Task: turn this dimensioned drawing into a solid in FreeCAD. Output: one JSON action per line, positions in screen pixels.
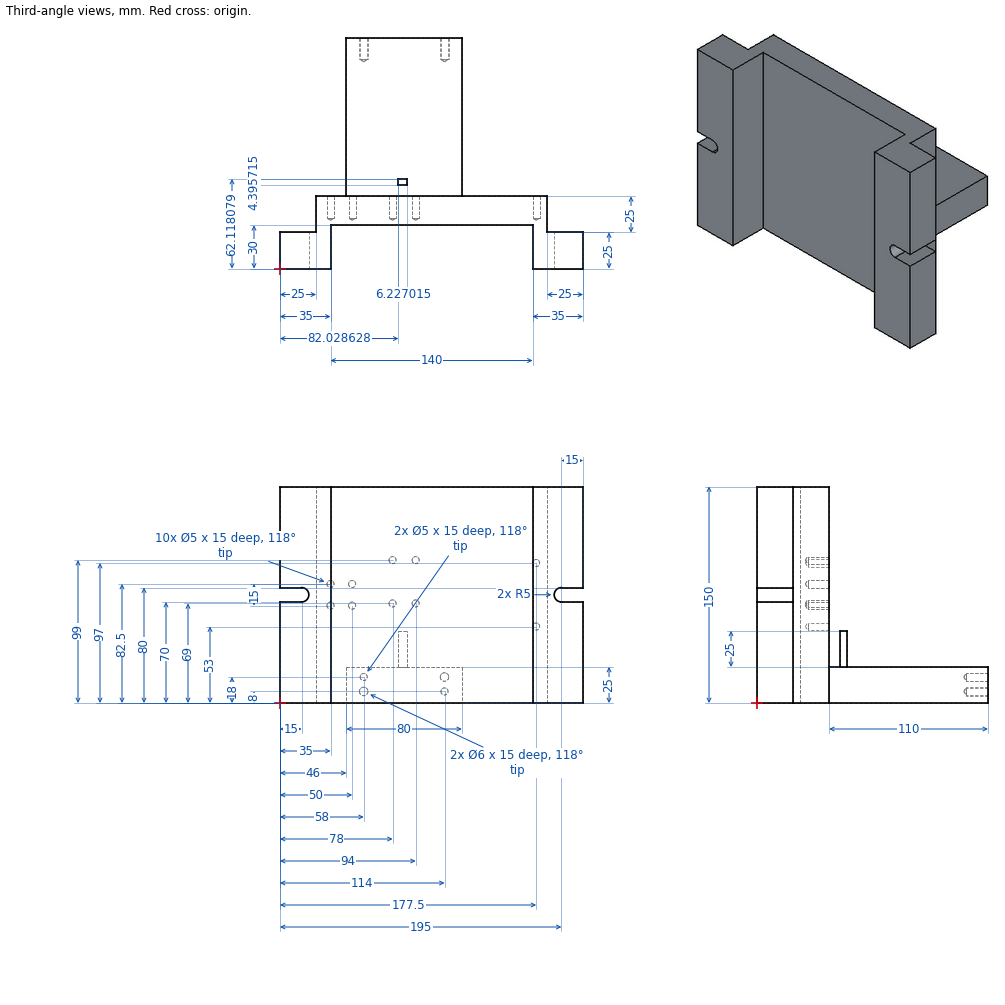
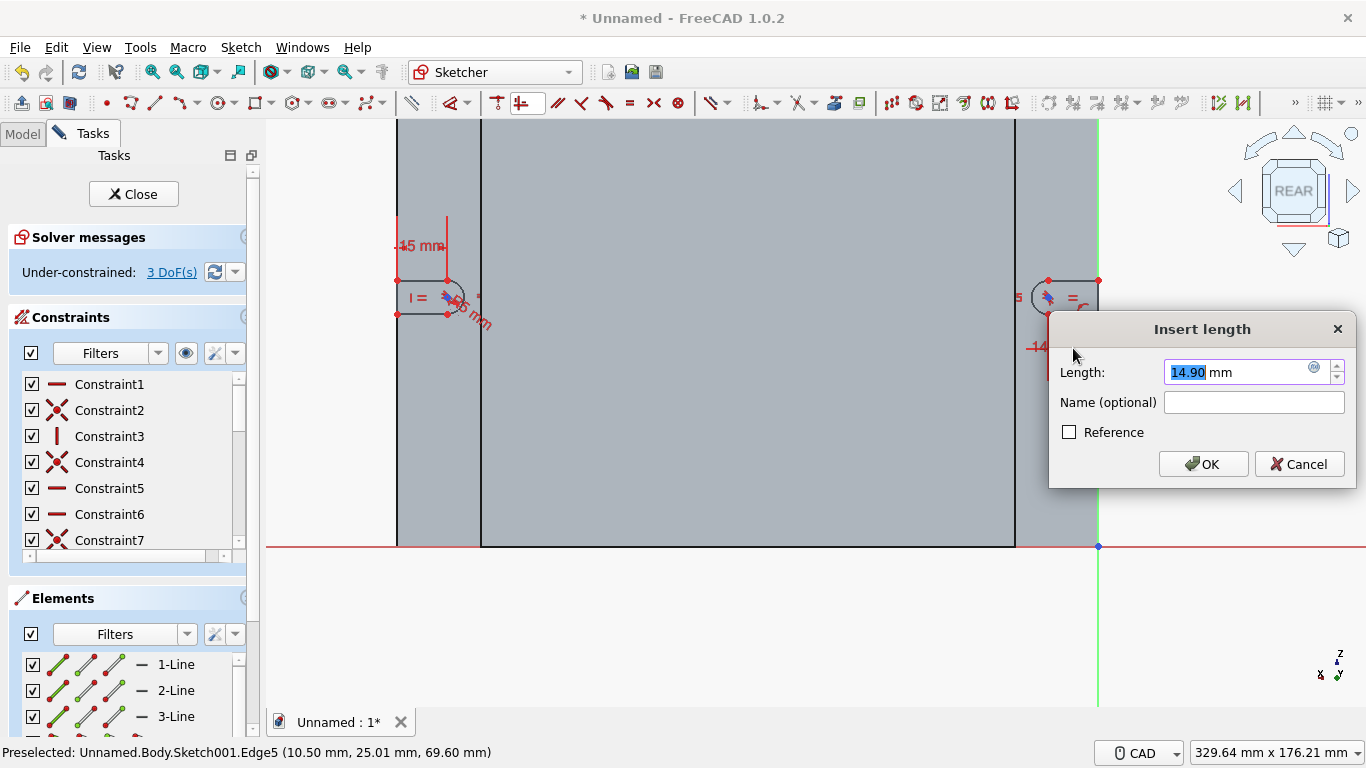
{"action": "type", "text": "15"}
{"action": "key", "text": "Return"}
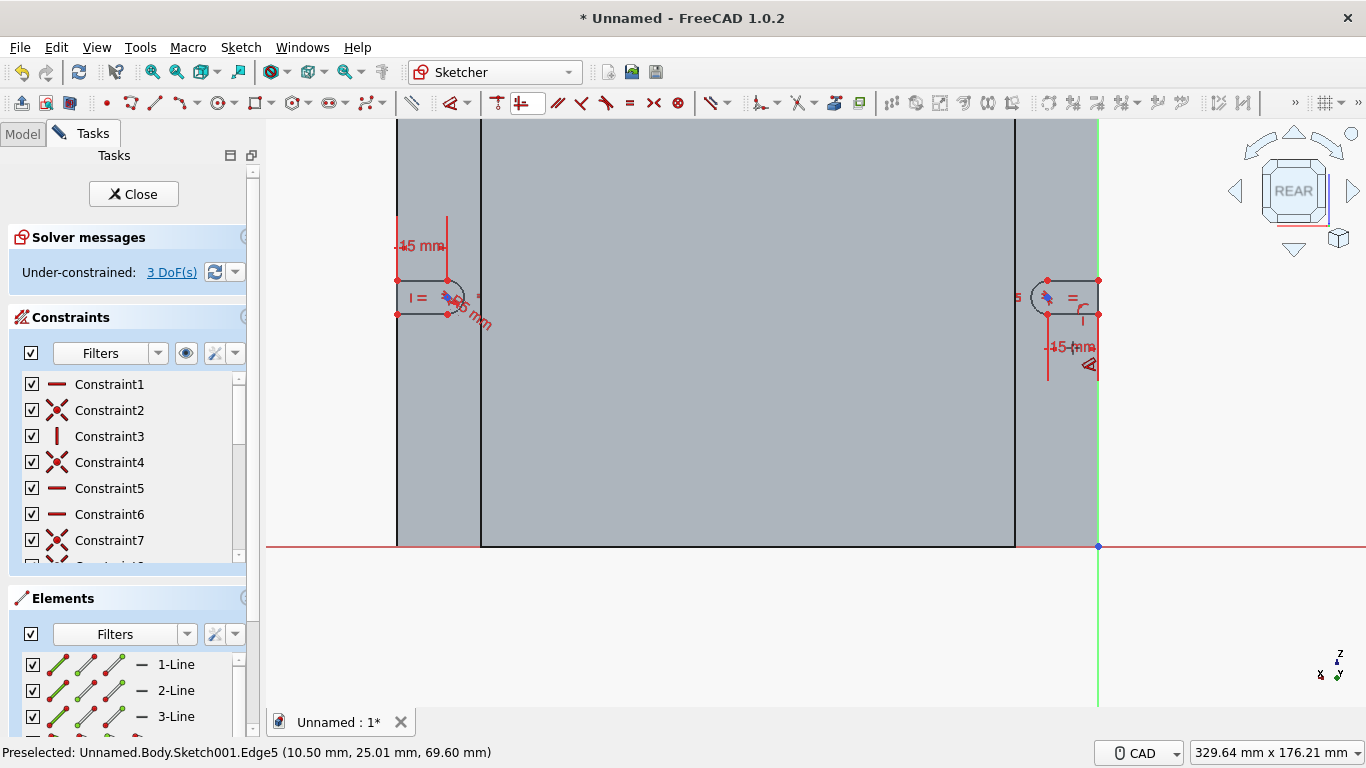
{"action": "left_click", "coordinate": [447, 281]}
{"action": "left_click", "coordinate": [1132, 414]}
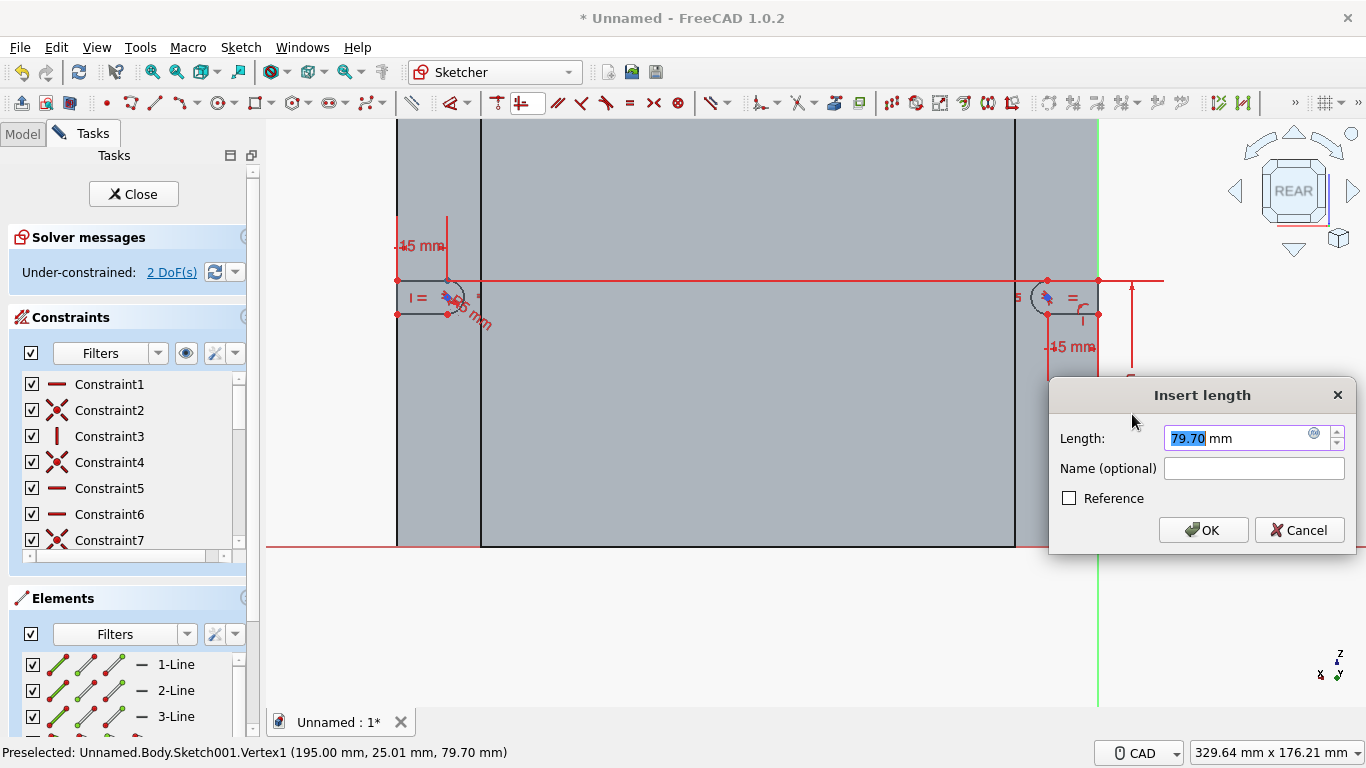
{"action": "type", "text": "80"}
{"action": "key", "text": "Return"}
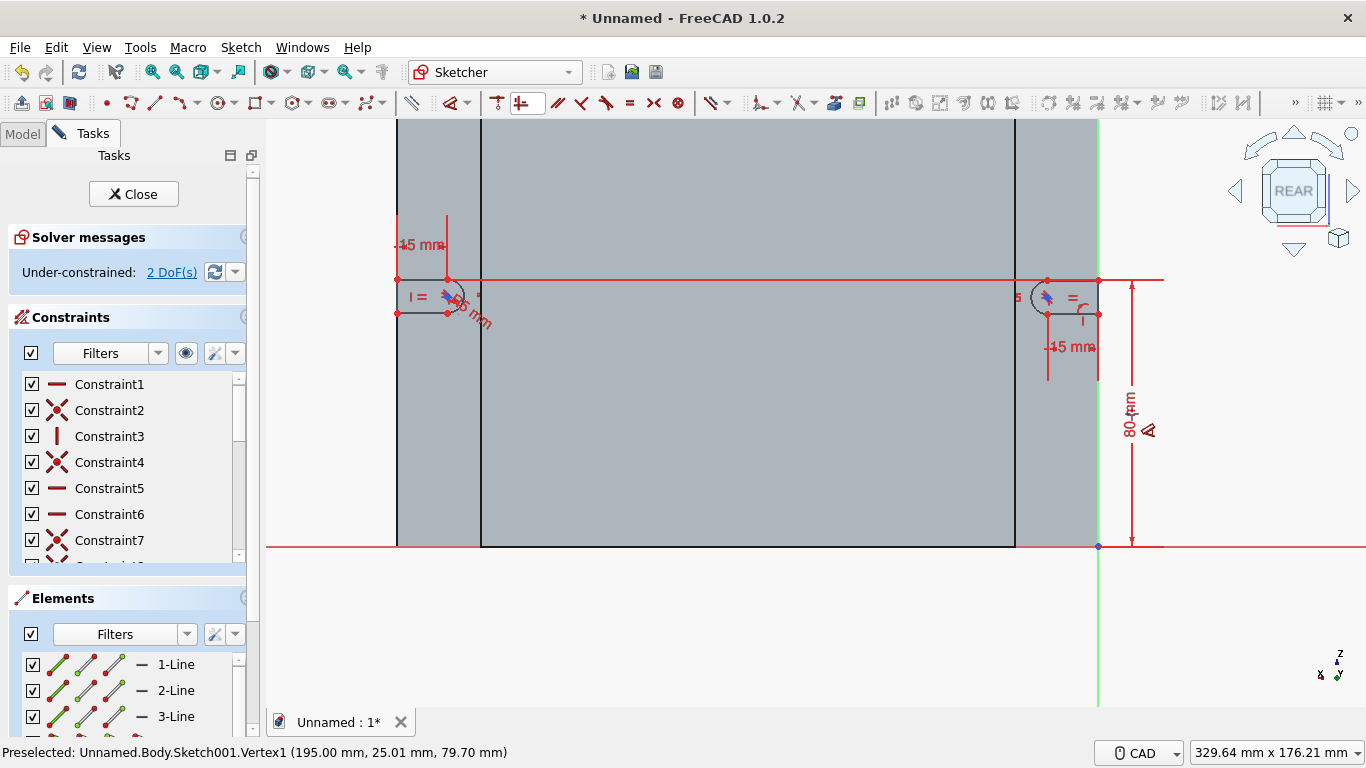
{"action": "left_click", "coordinate": [1048, 314]}
{"action": "left_click", "coordinate": [1132, 377]}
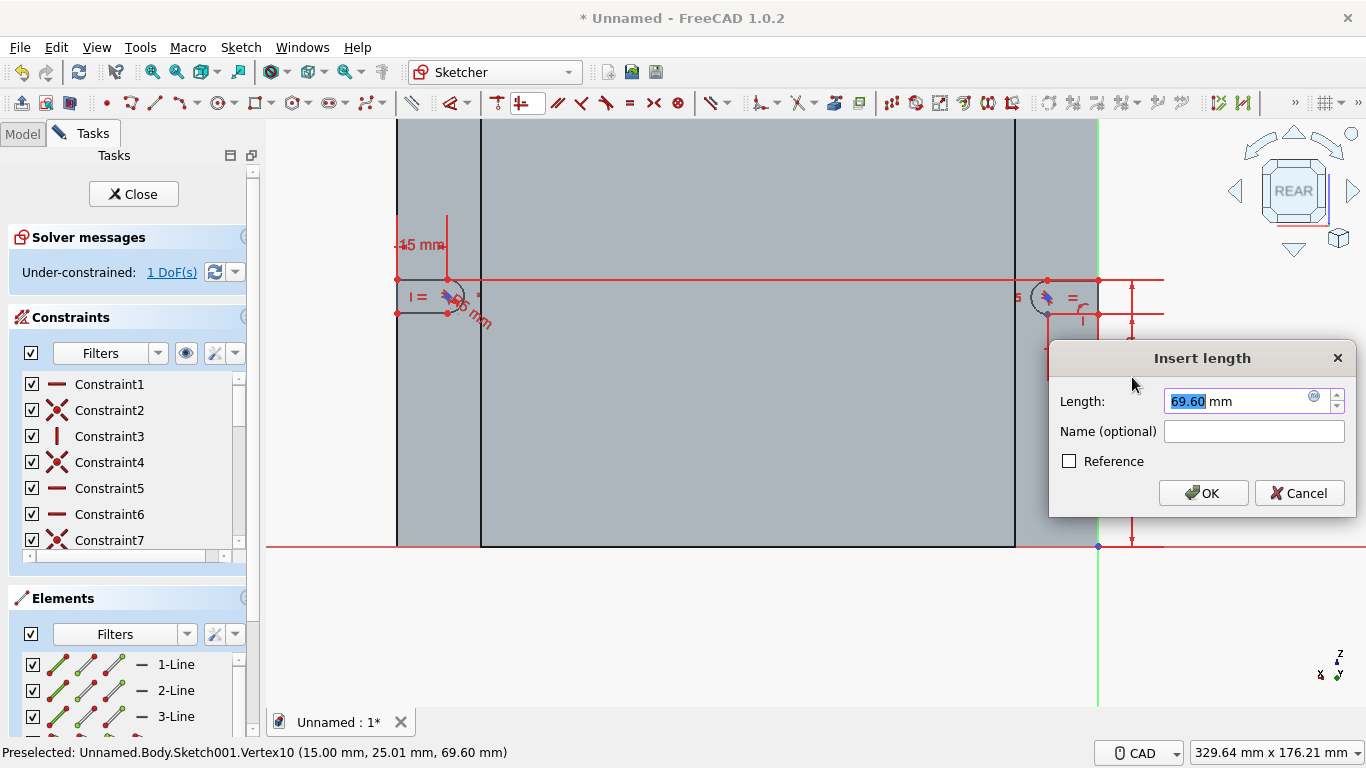
{"action": "type", "text": "70"}
{"action": "key", "text": "Return"}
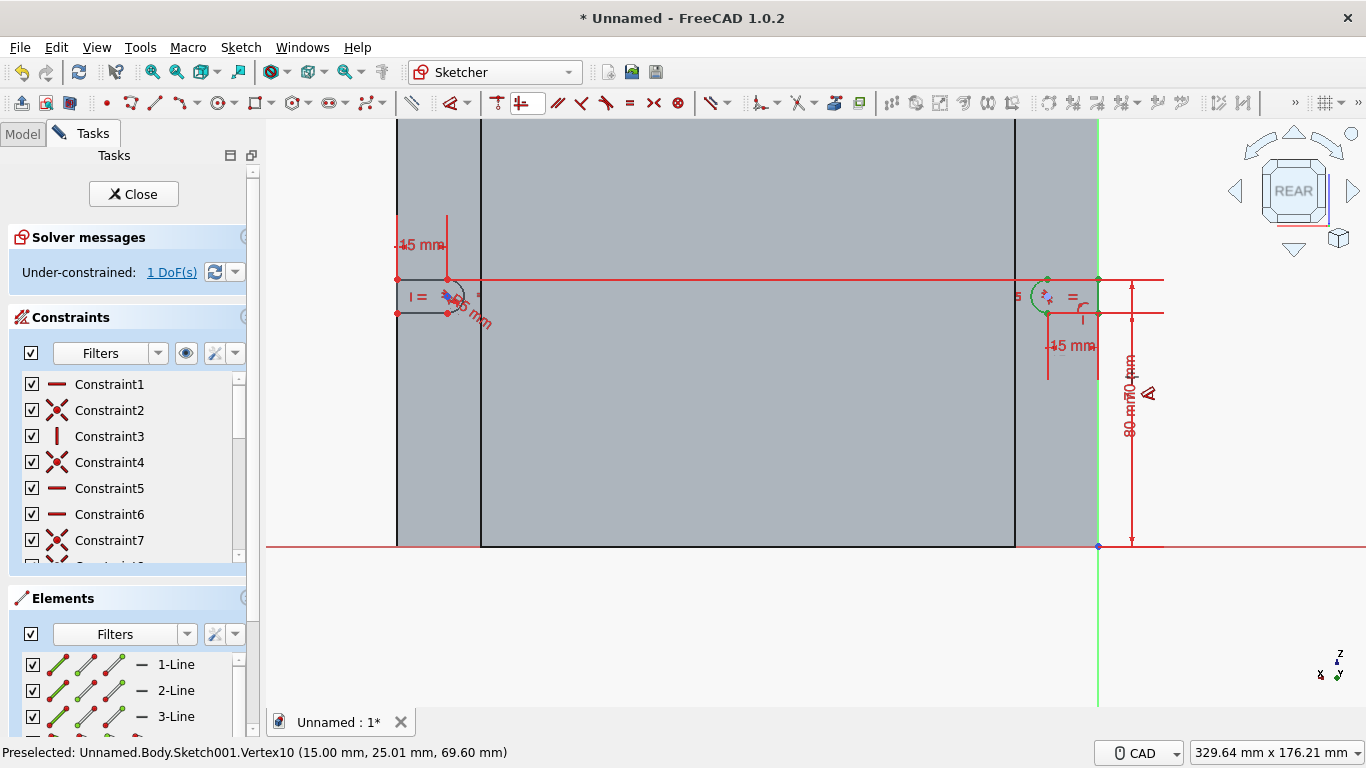
{"action": "left_click", "coordinate": [447, 280]}
{"action": "left_click", "coordinate": [773, 581]}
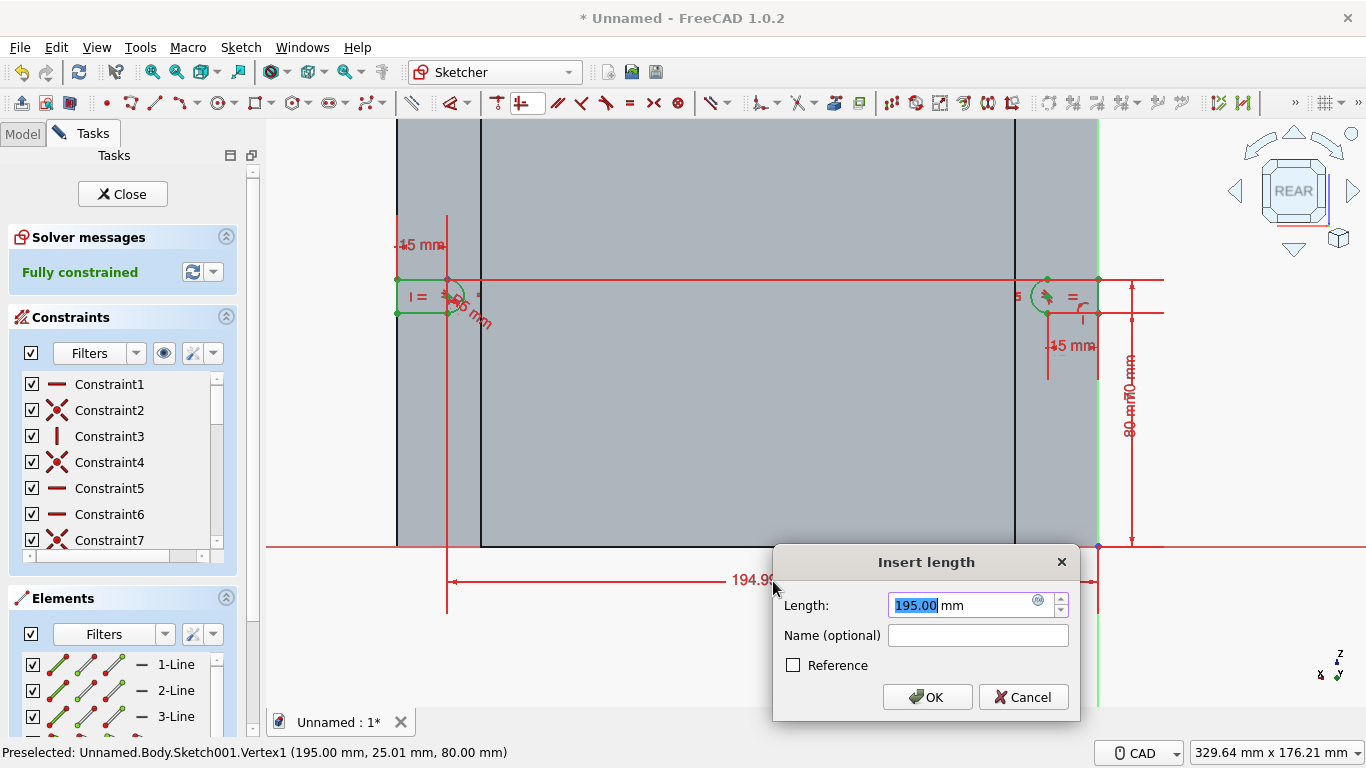
{"action": "type", "text": "195"}
{"action": "key", "text": "Return"}
{"action": "key", "text": "Escape"}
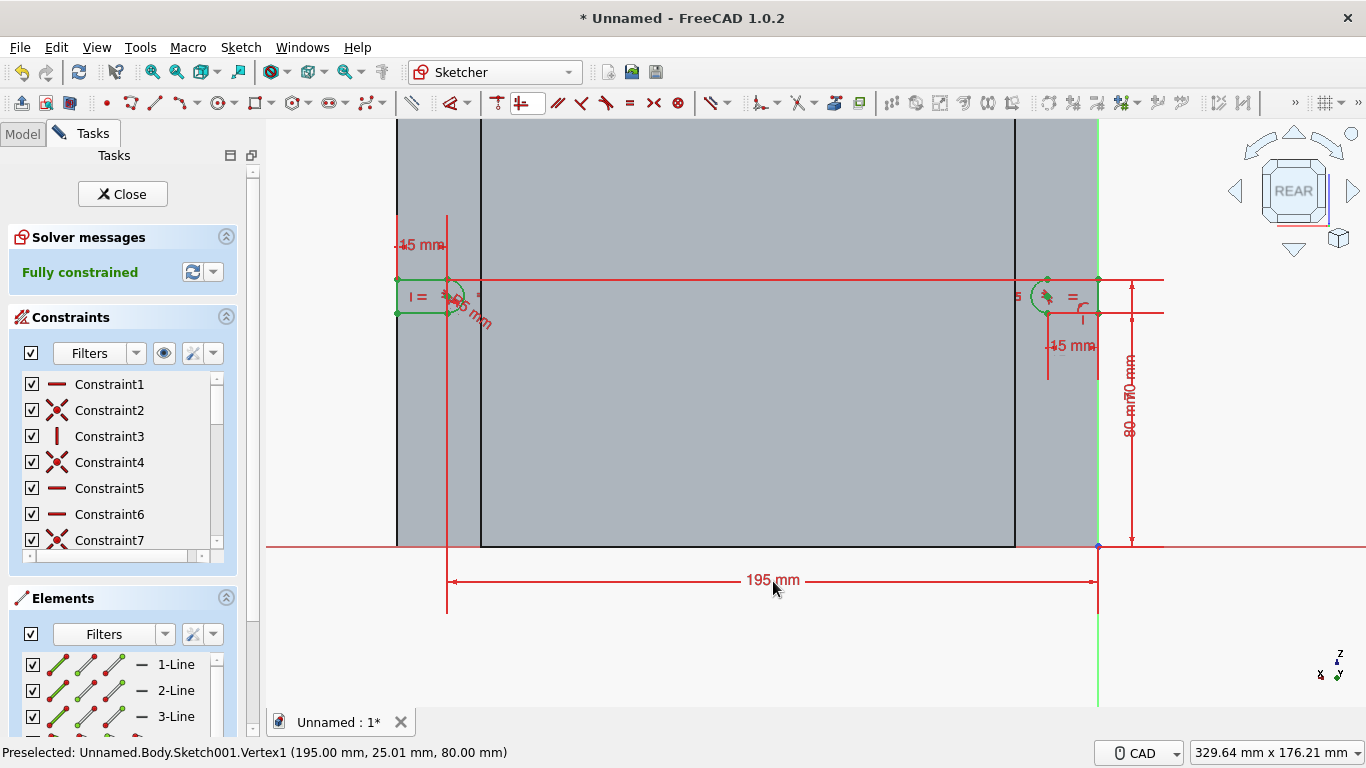
{"action": "left_click", "coordinate": [123, 194]}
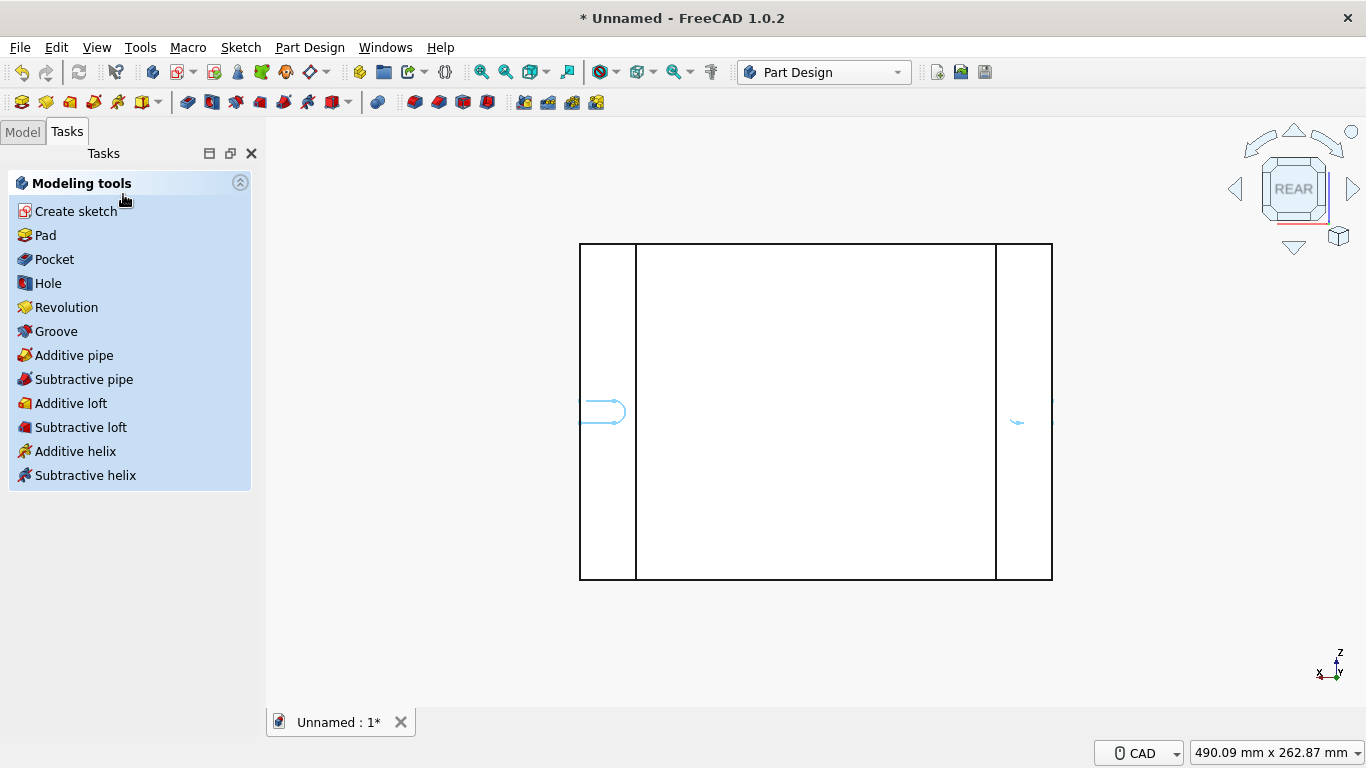
{"action": "left_click", "coordinate": [188, 102]}